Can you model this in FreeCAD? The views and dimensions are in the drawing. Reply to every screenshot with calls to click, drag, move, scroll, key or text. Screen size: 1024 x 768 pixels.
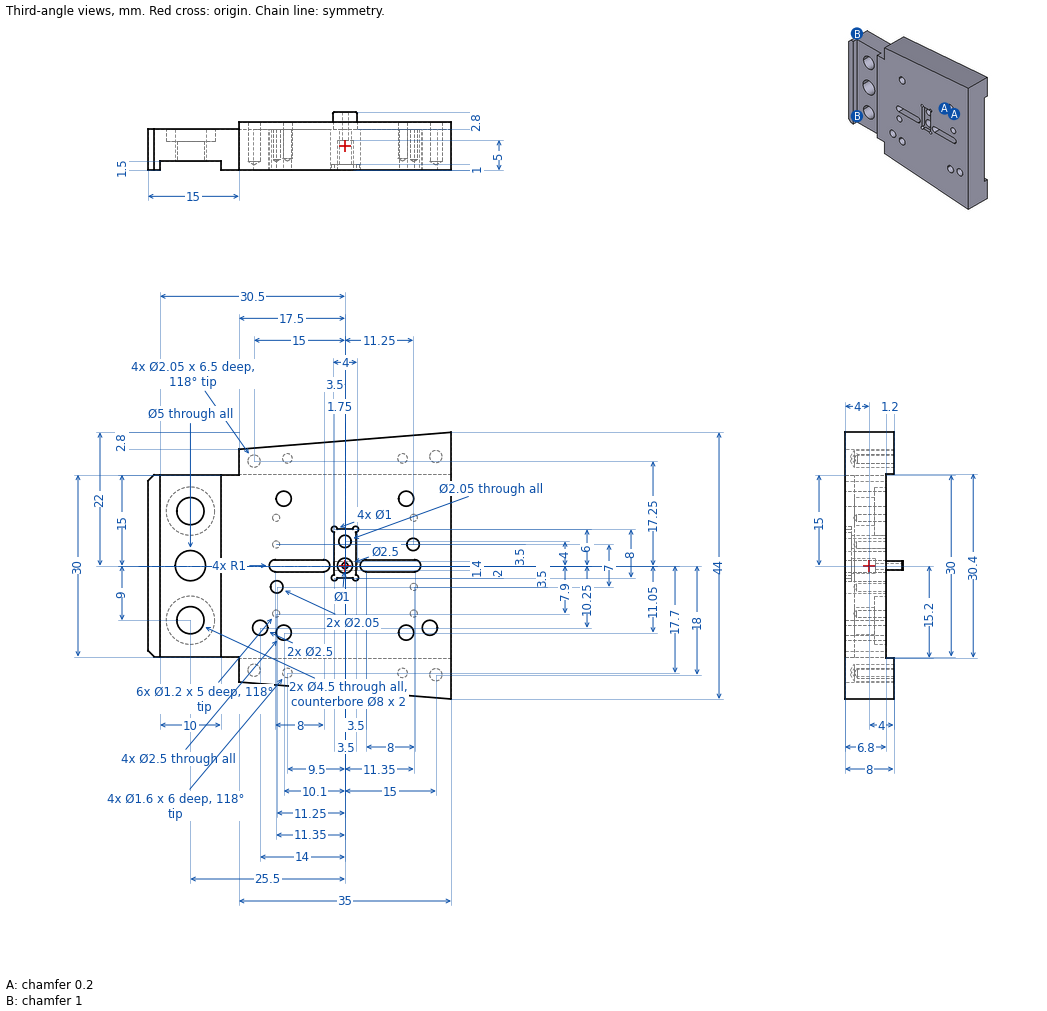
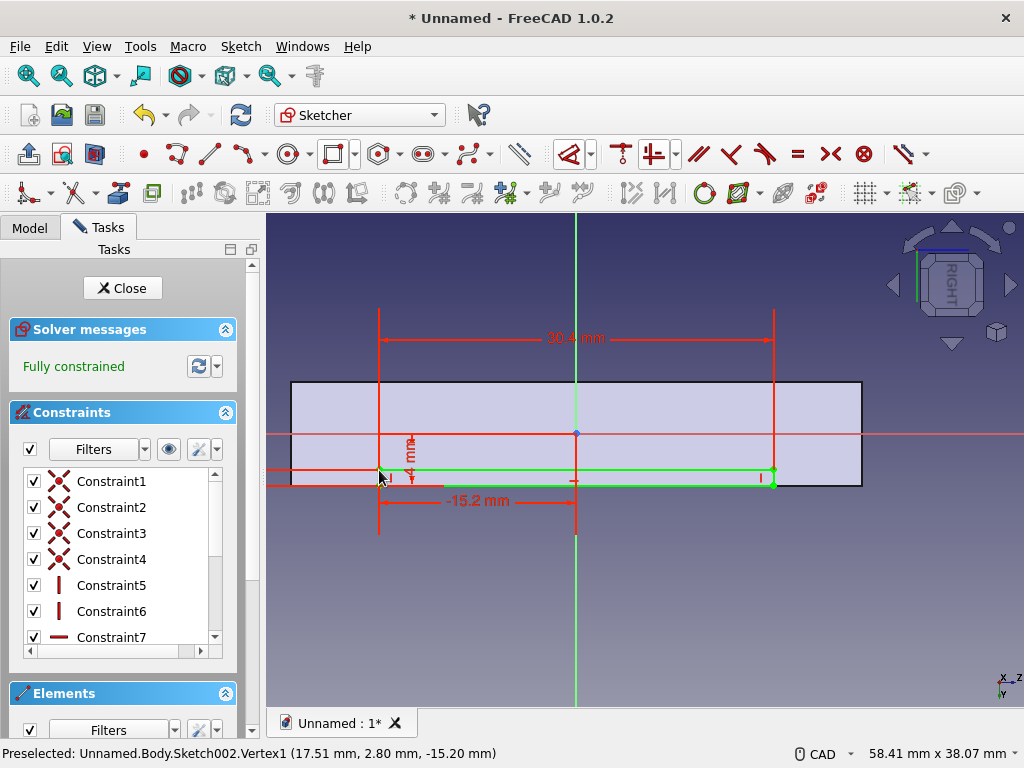
click(123, 288)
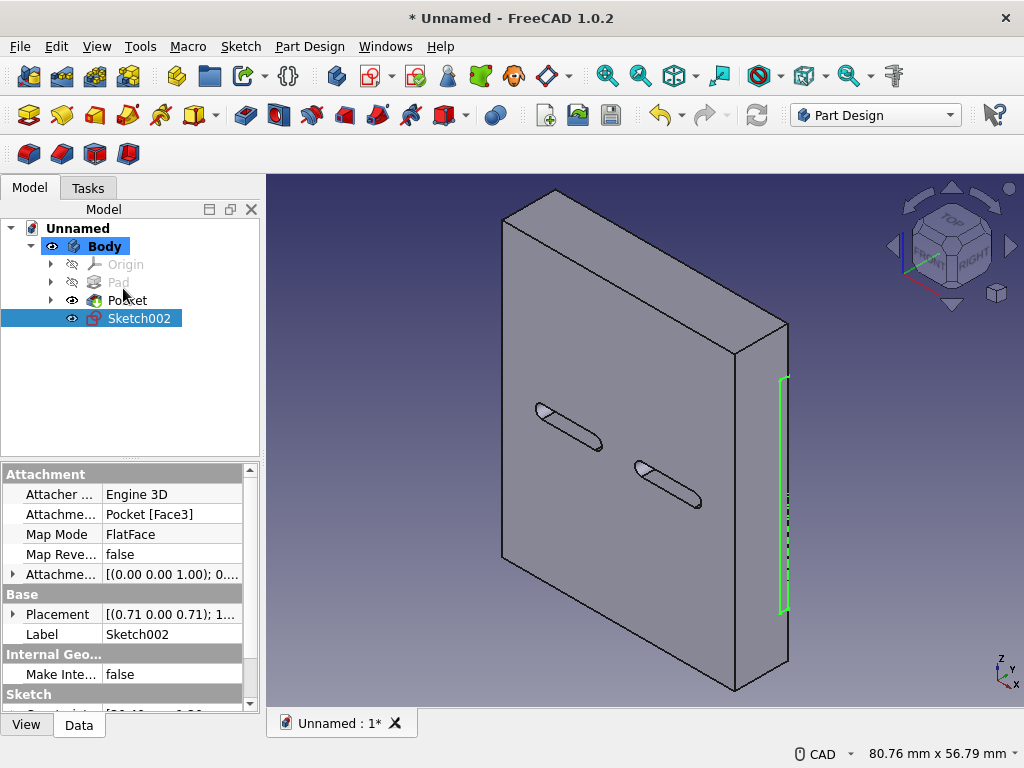
click(246, 116)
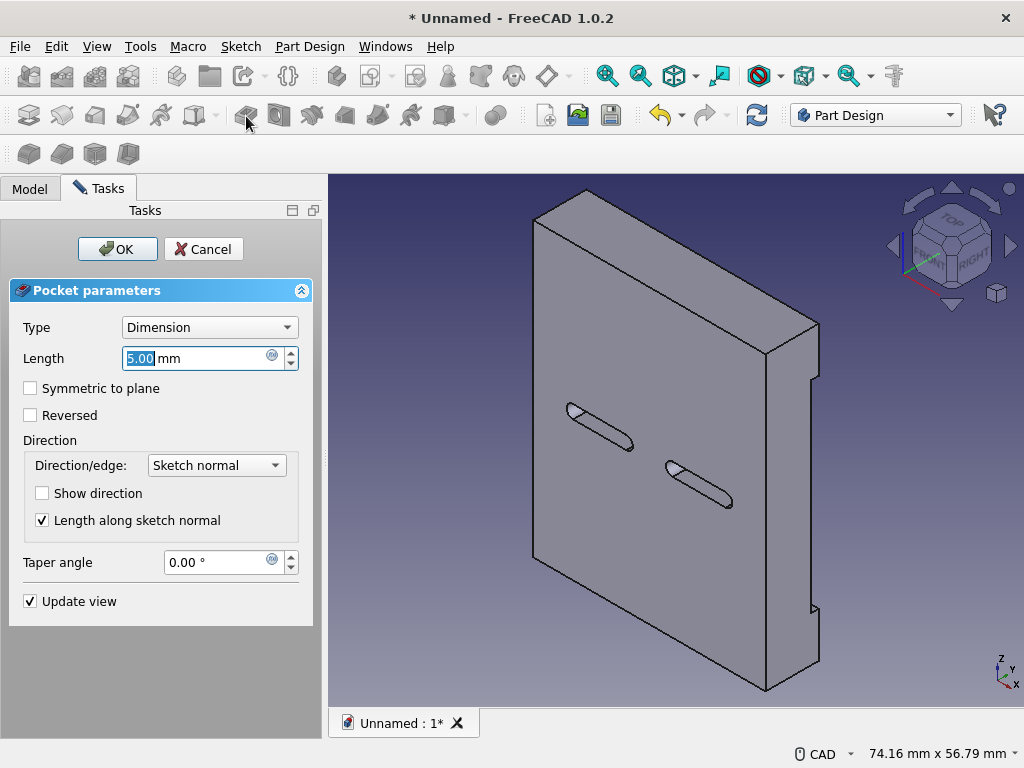
click(210, 328)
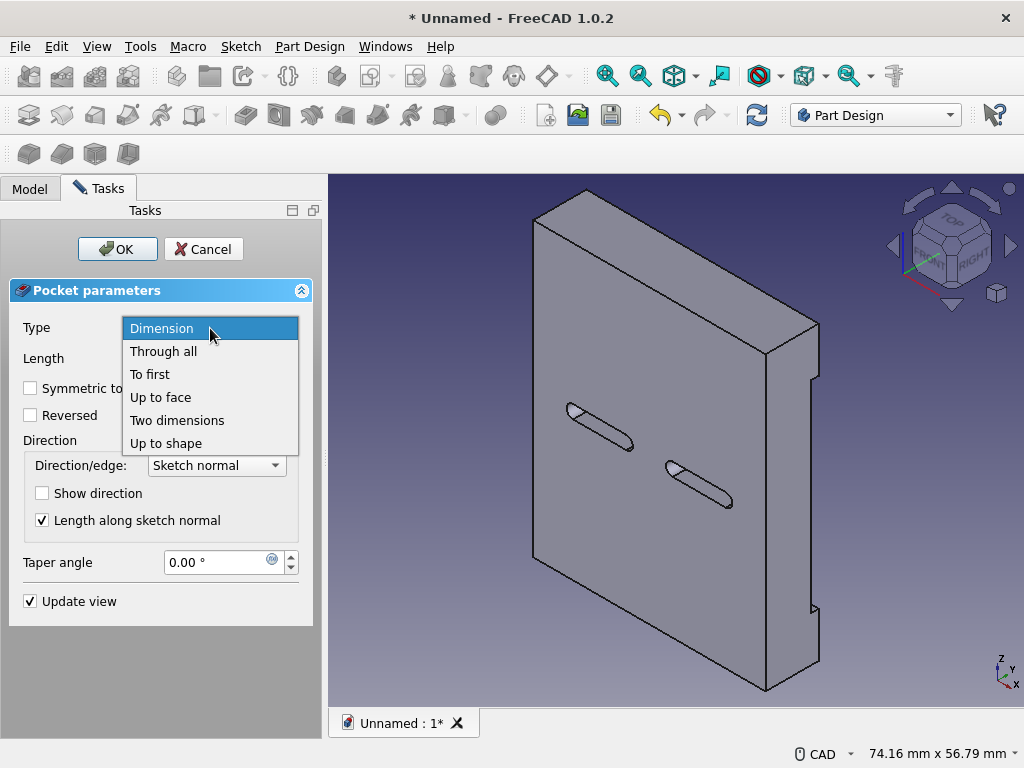
click(208, 352)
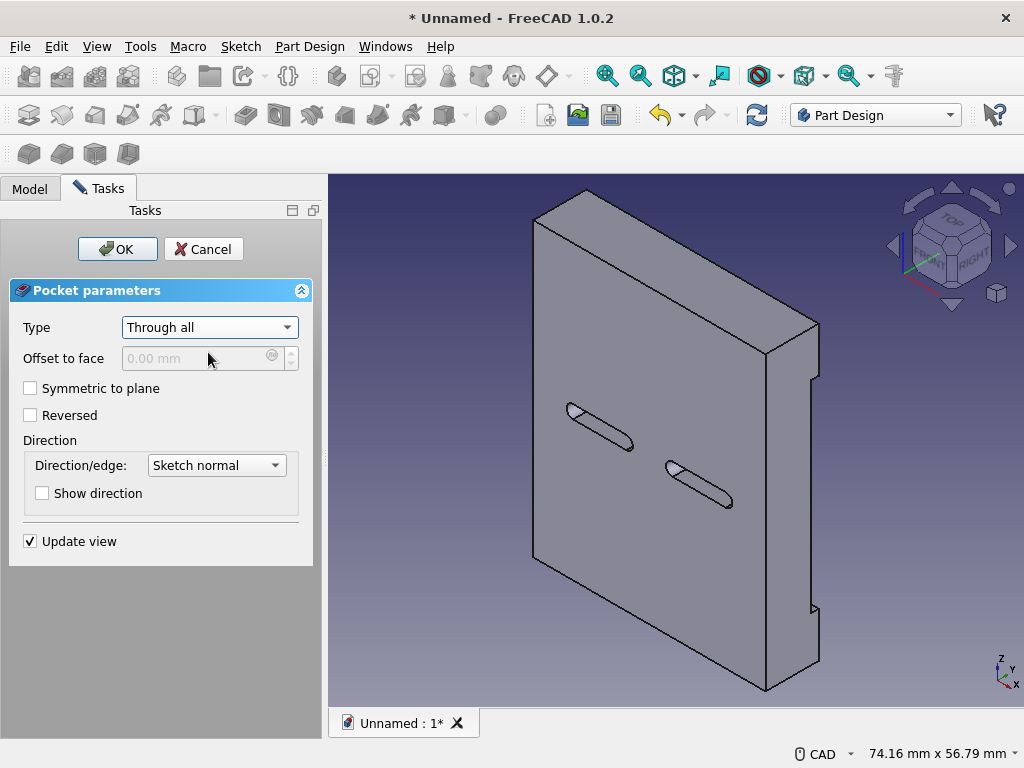
click(118, 249)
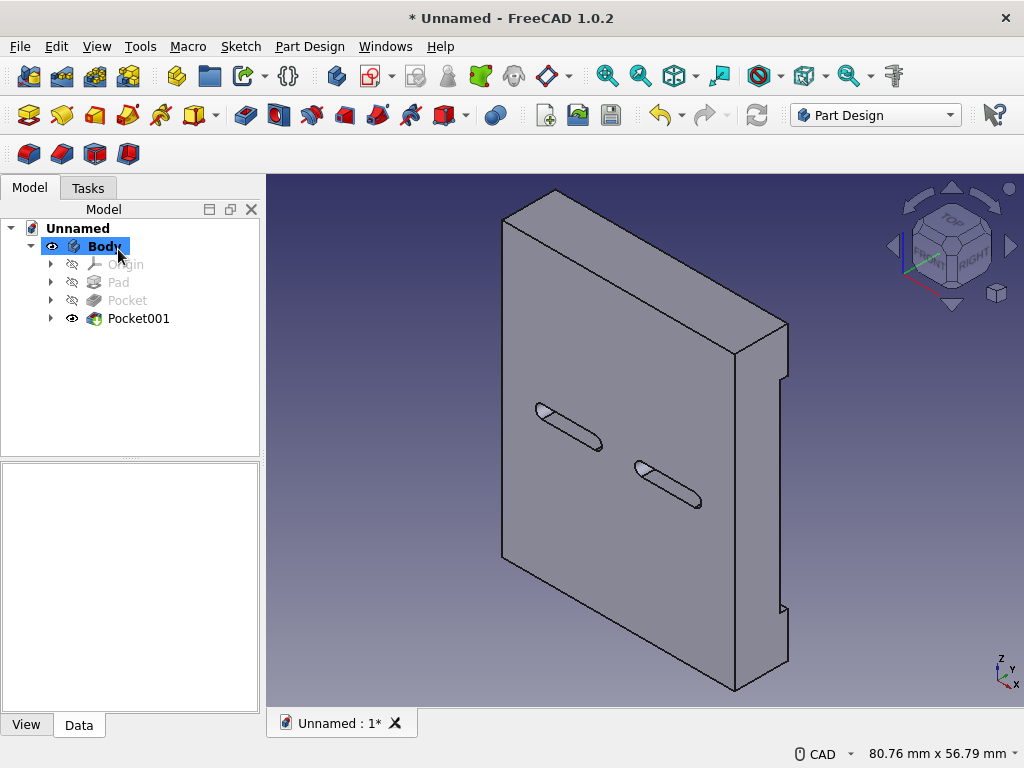
key(4)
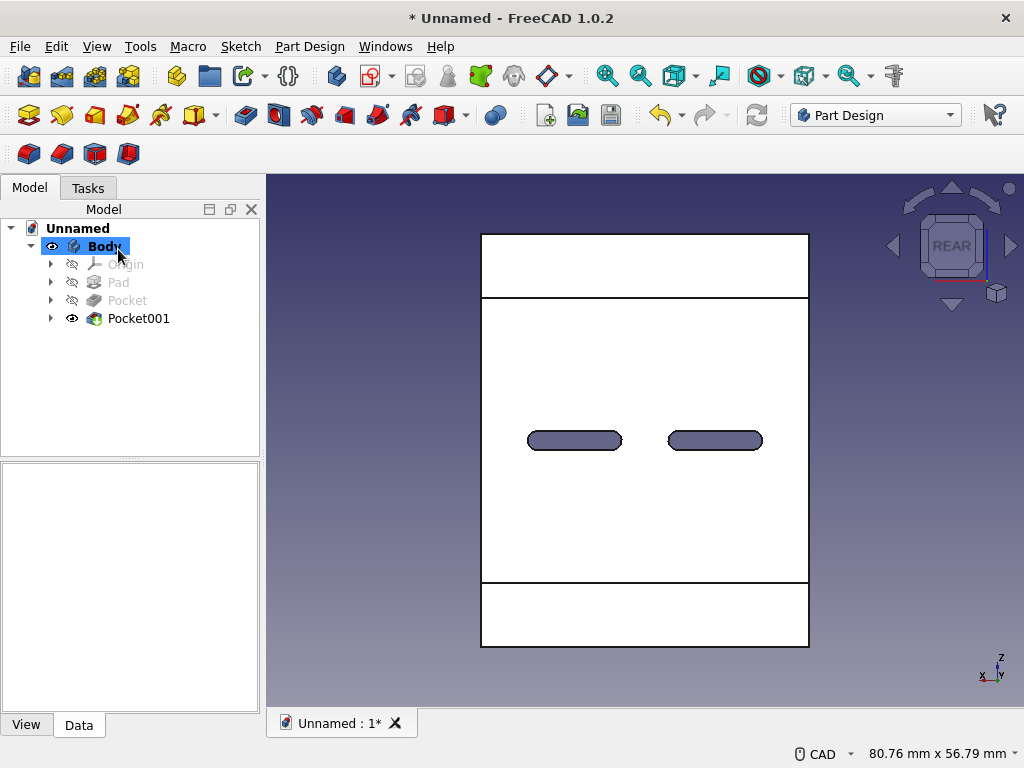
click(739, 521)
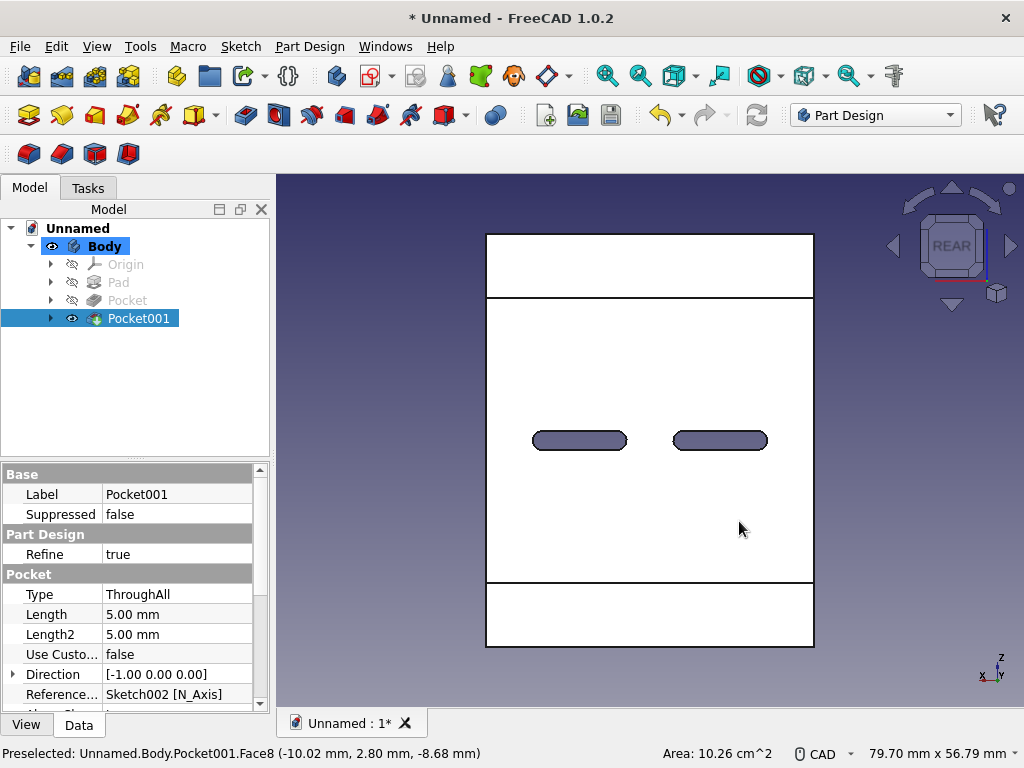
click(370, 76)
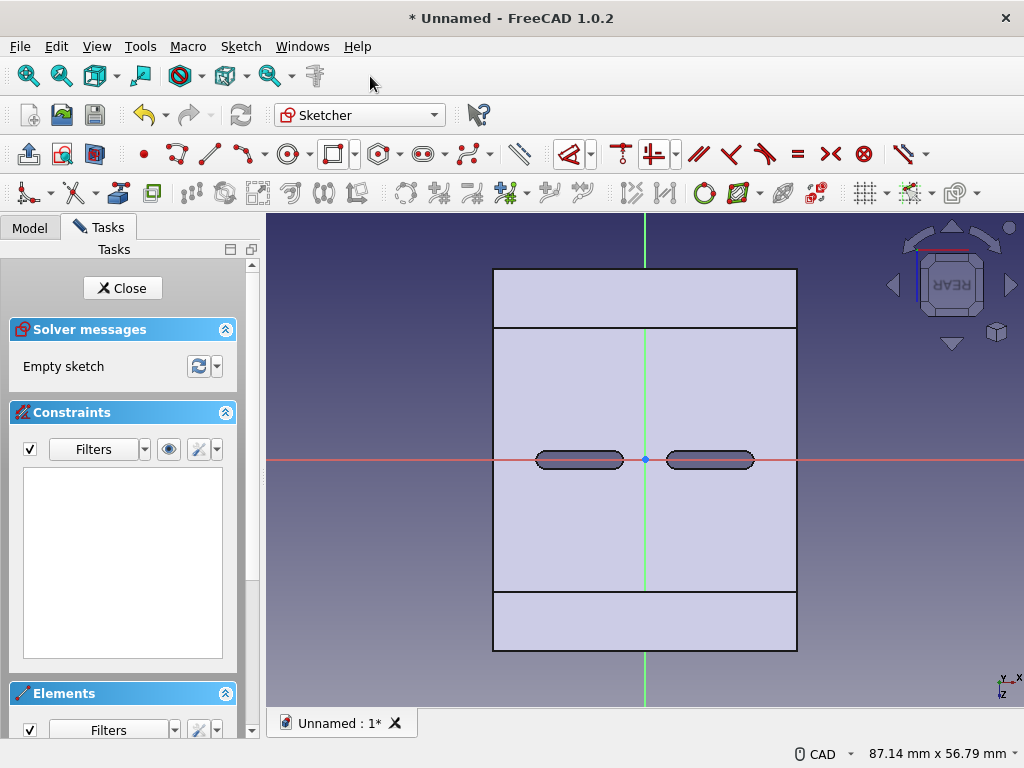
click(95, 154)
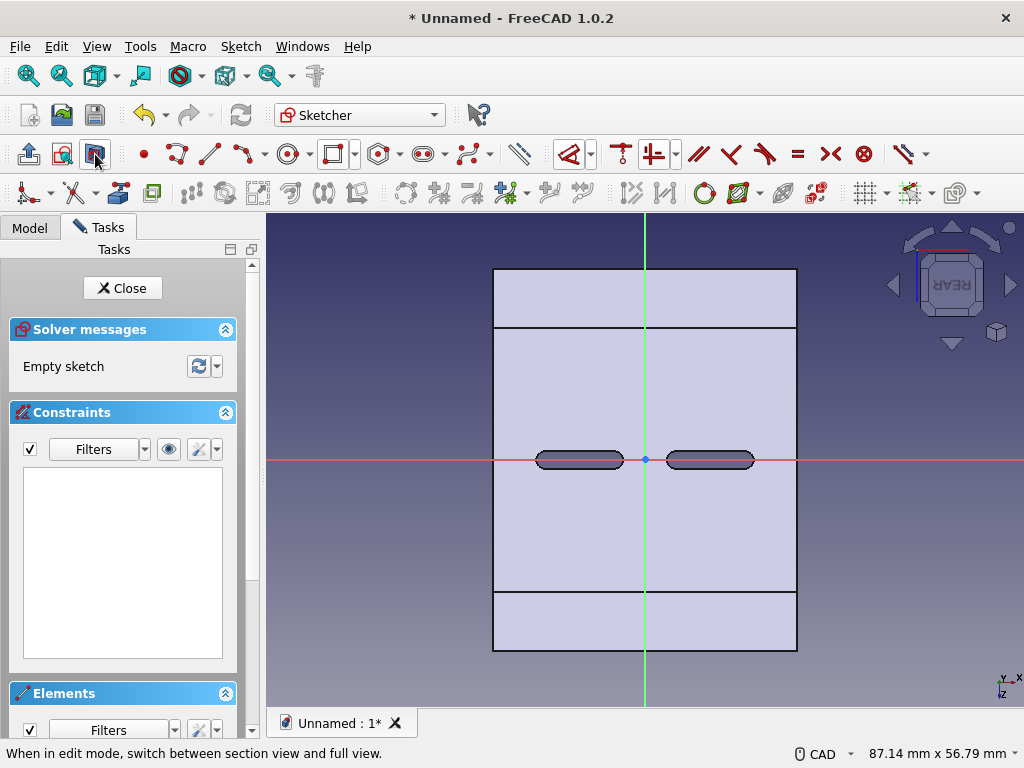
scroll(652, 460, up, 12)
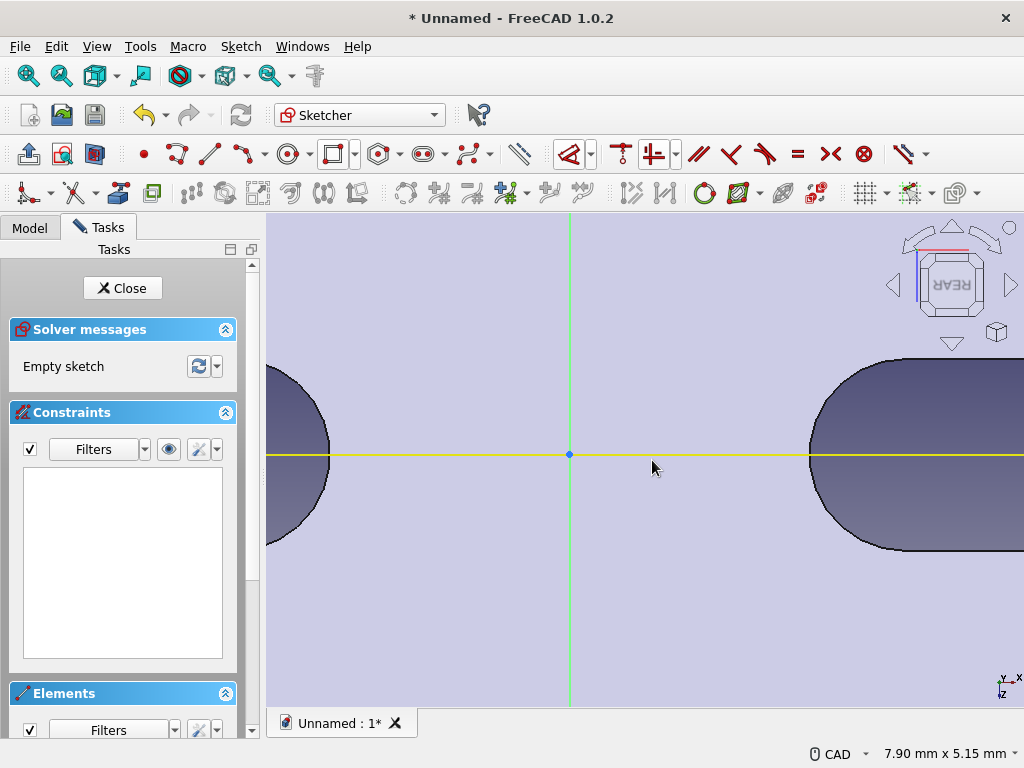
click(354, 154)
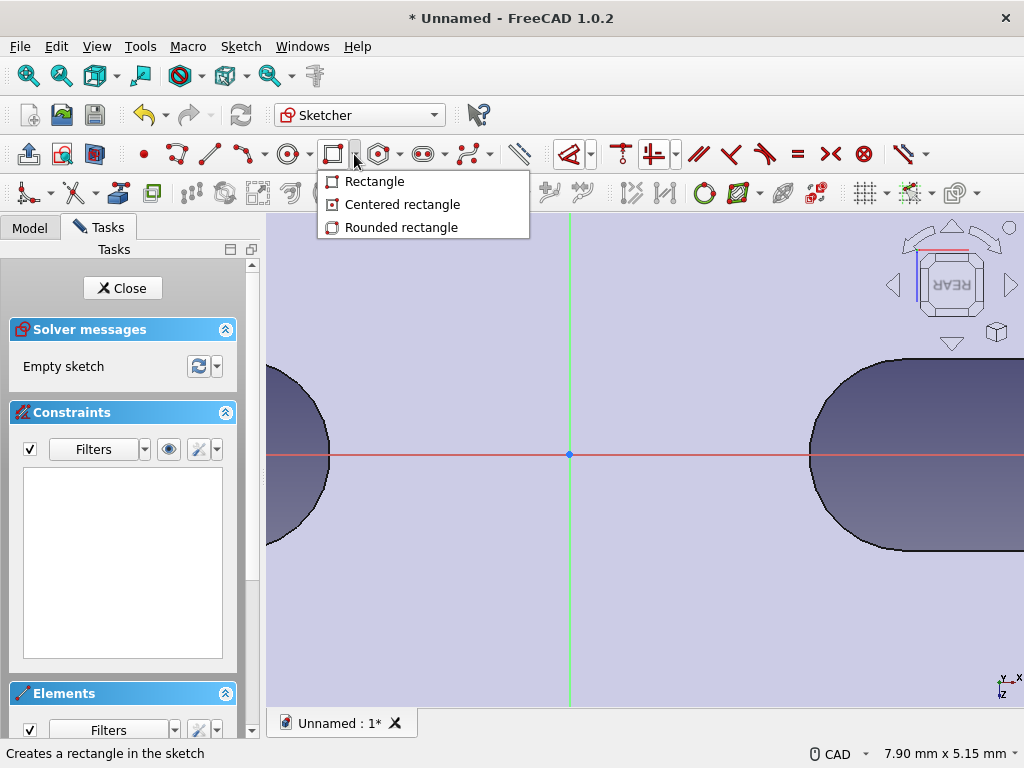
click(424, 204)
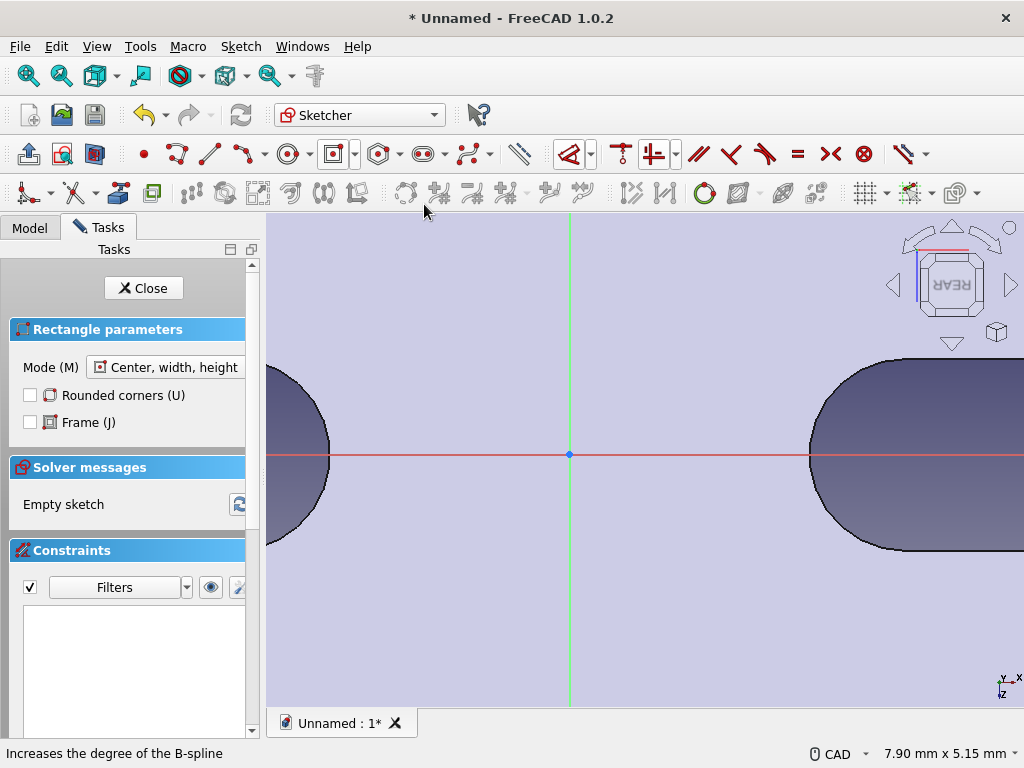
click(570, 455)
move(762, 388)